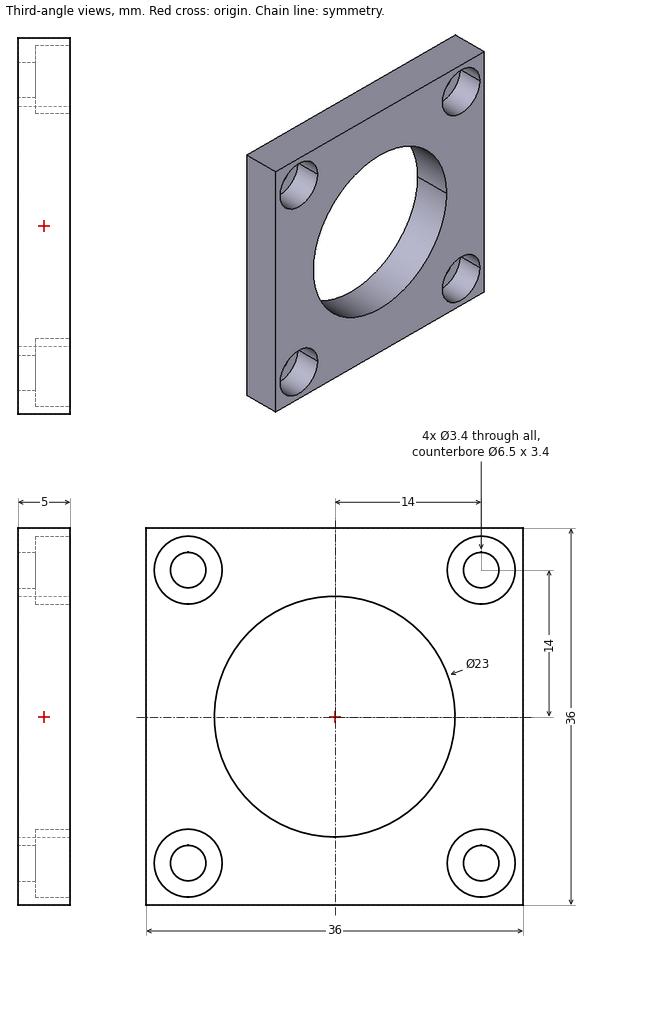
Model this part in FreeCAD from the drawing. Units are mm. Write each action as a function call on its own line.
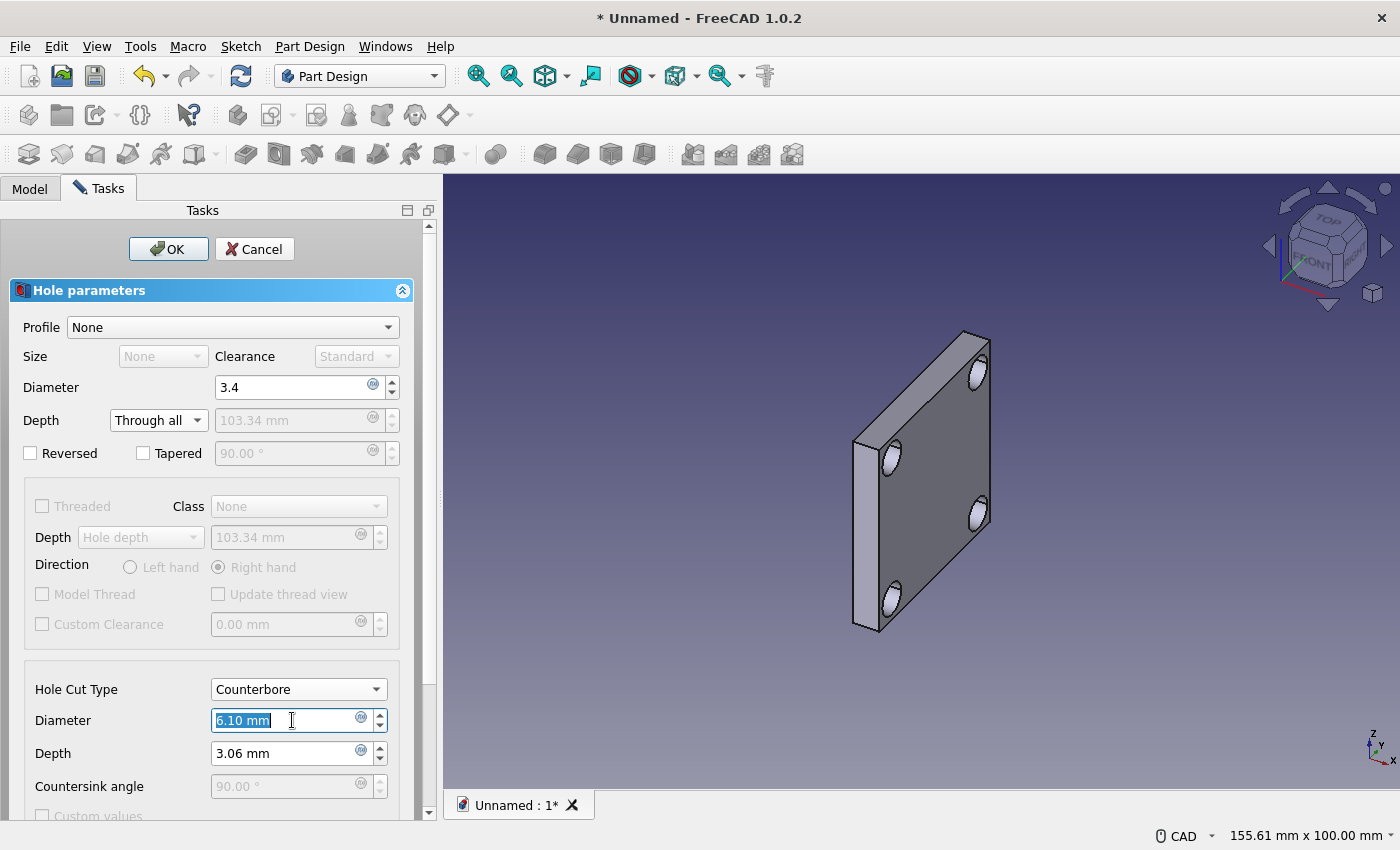
text(6.5)
key(Tab)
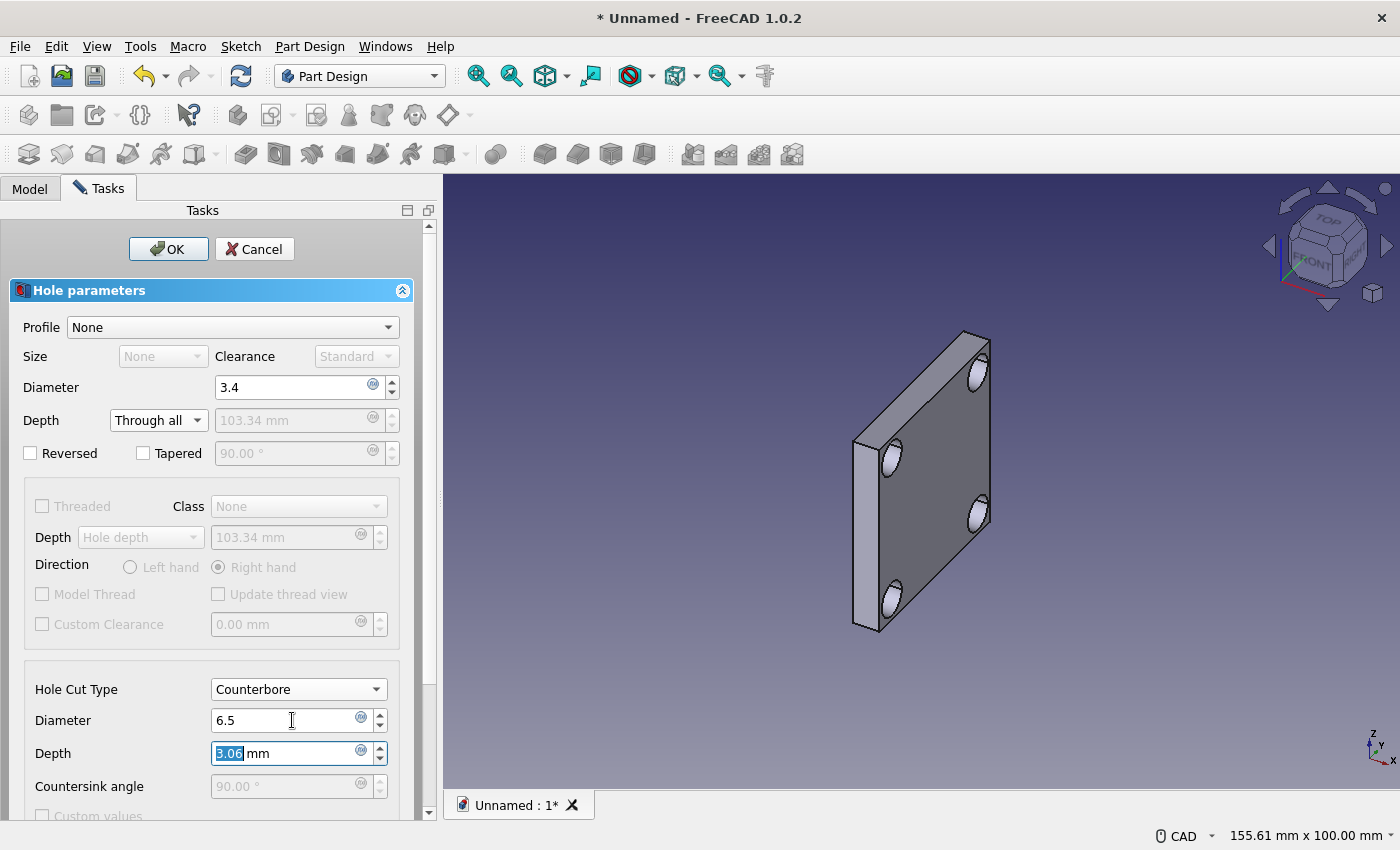
text(3.4)
key(Tab)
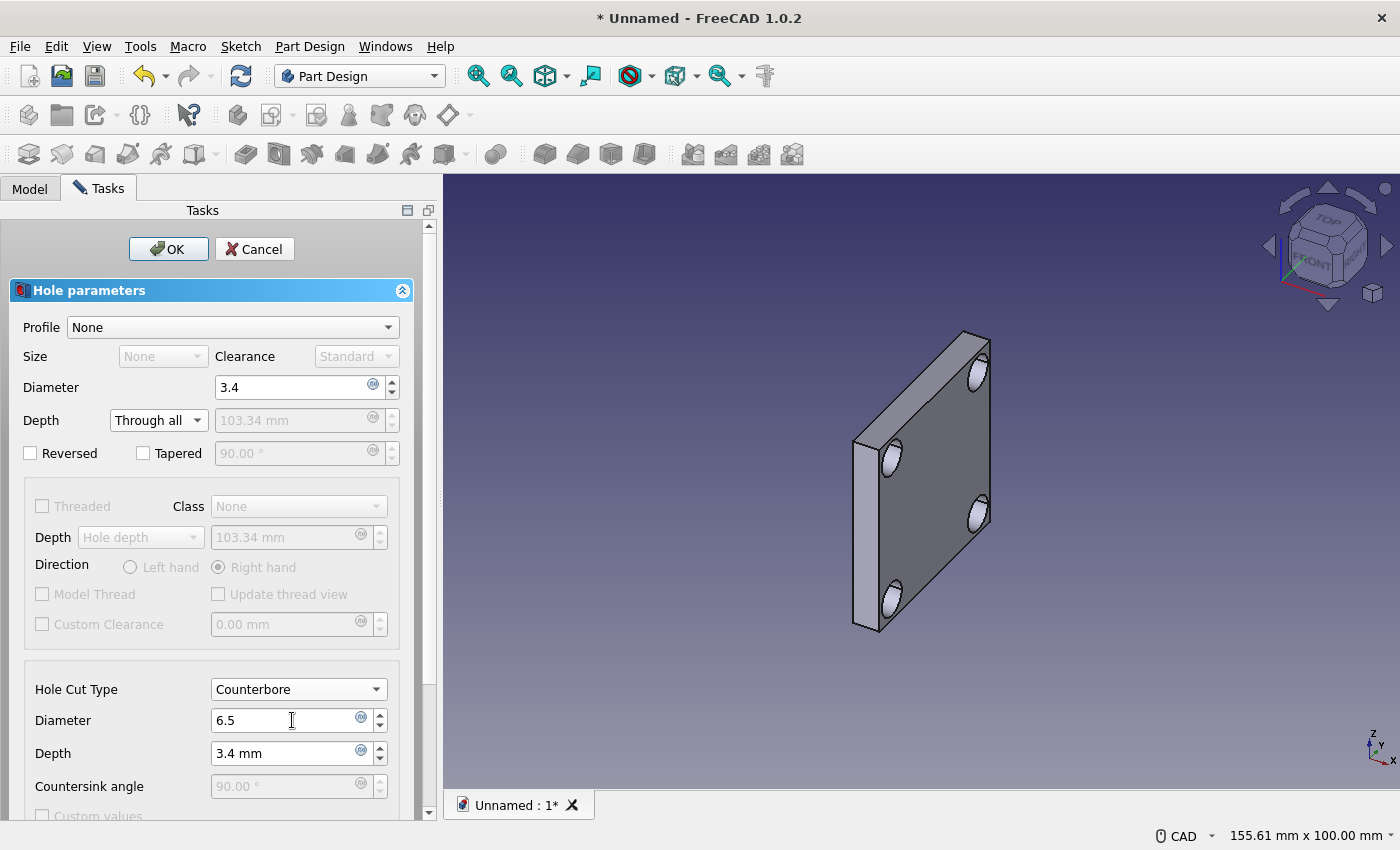
click(169, 249)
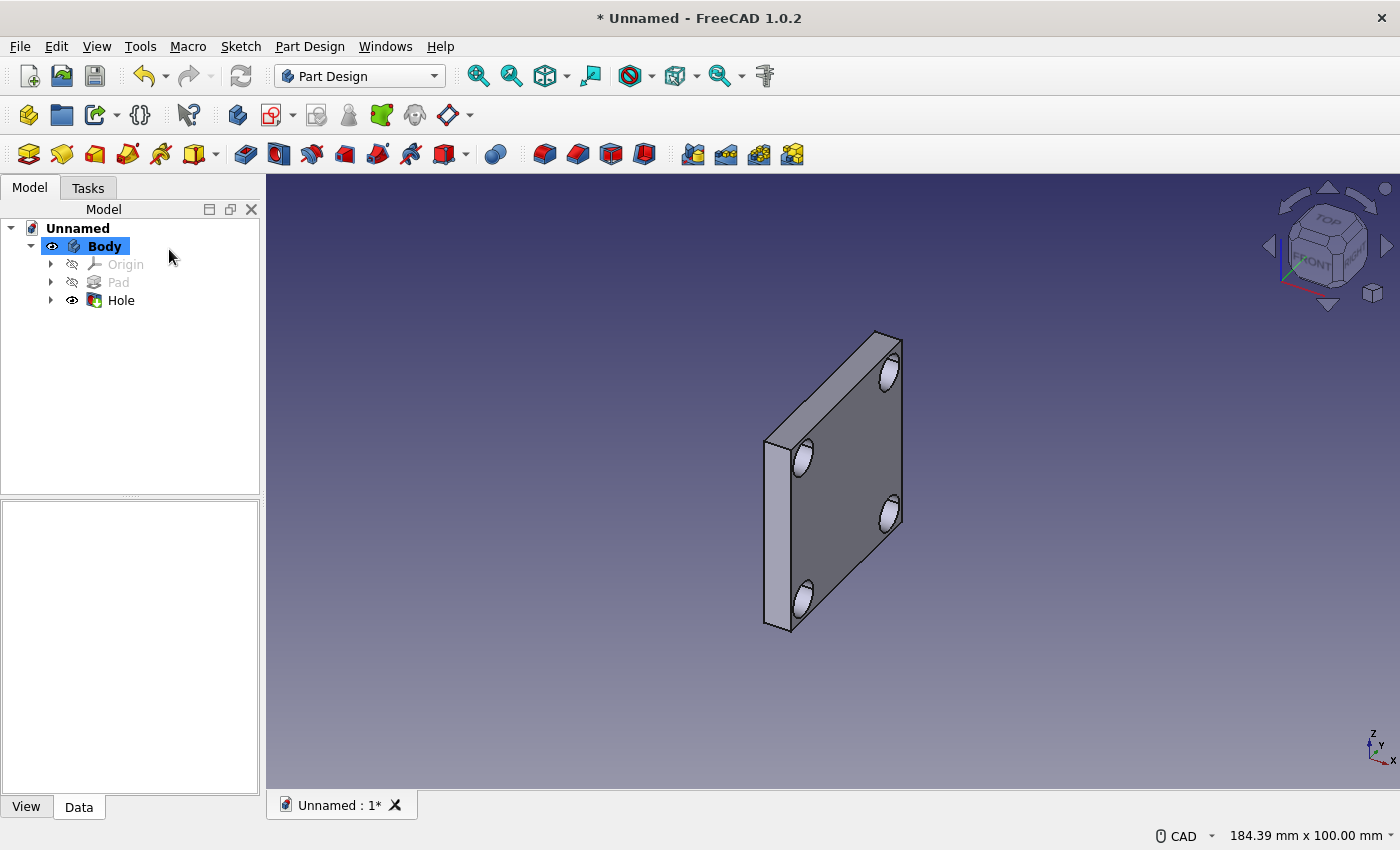
click(846, 485)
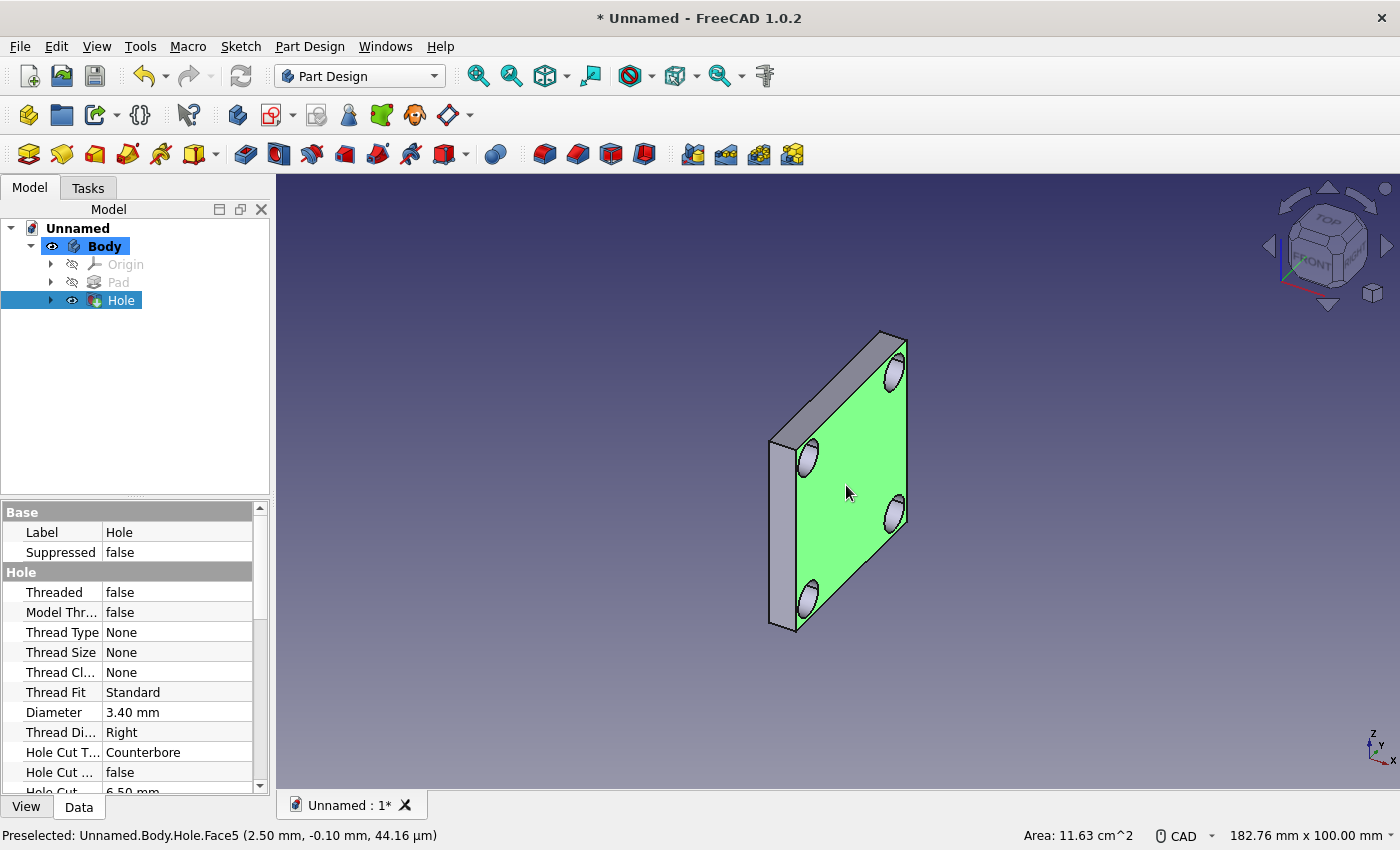
click(270, 116)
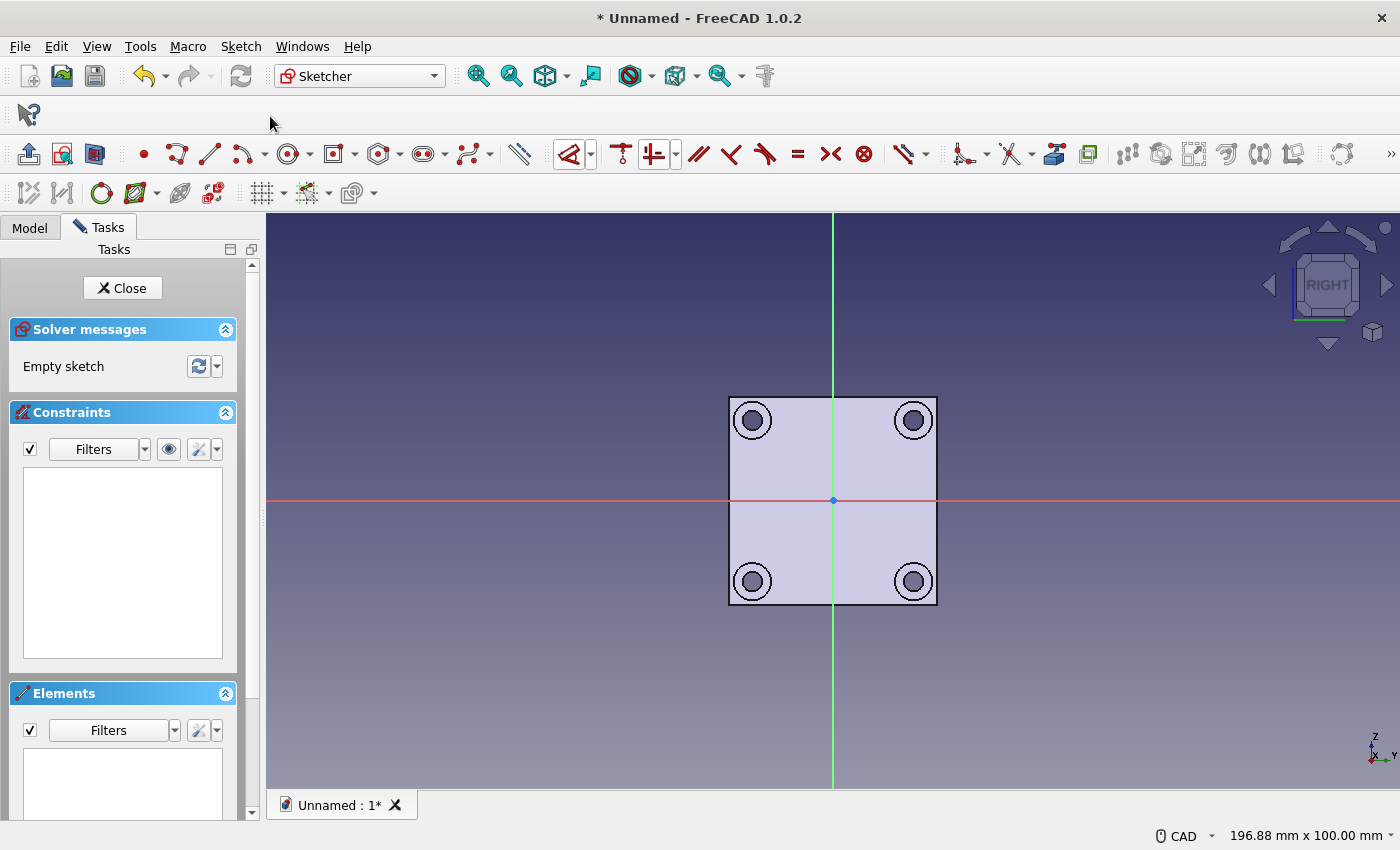
scroll(873, 501, up, 5)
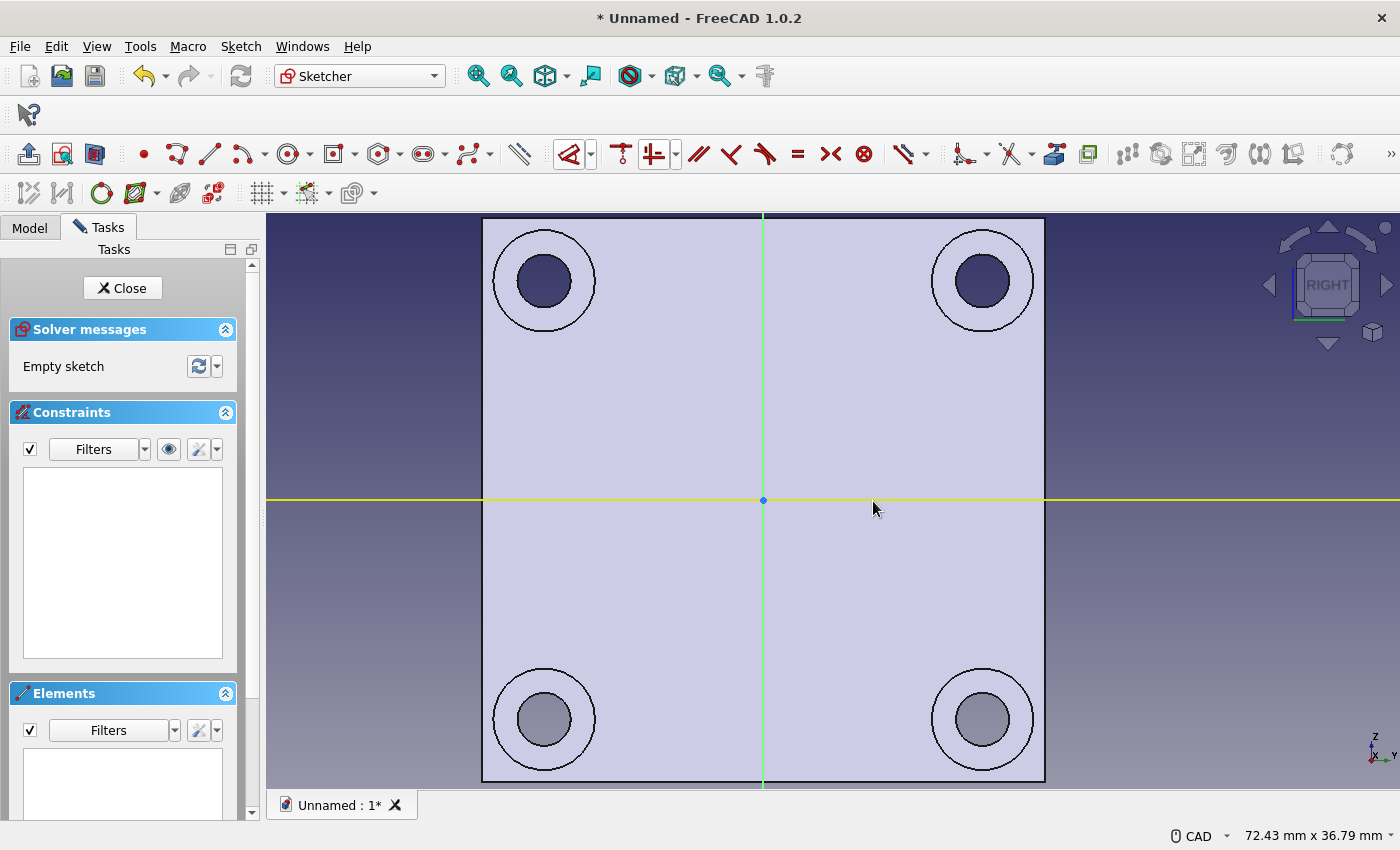
click(288, 154)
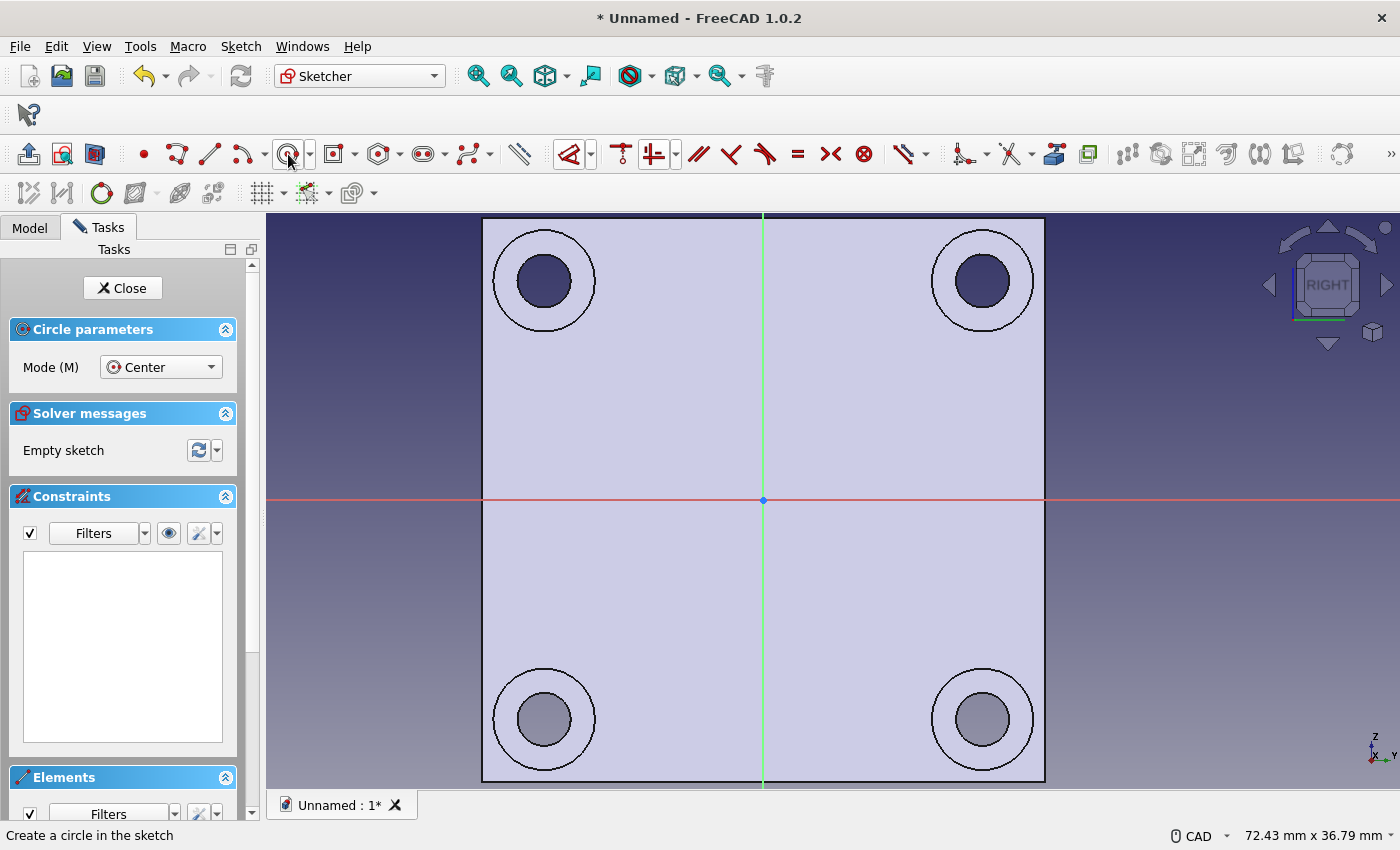
click(763, 500)
click(891, 373)
key(Escape)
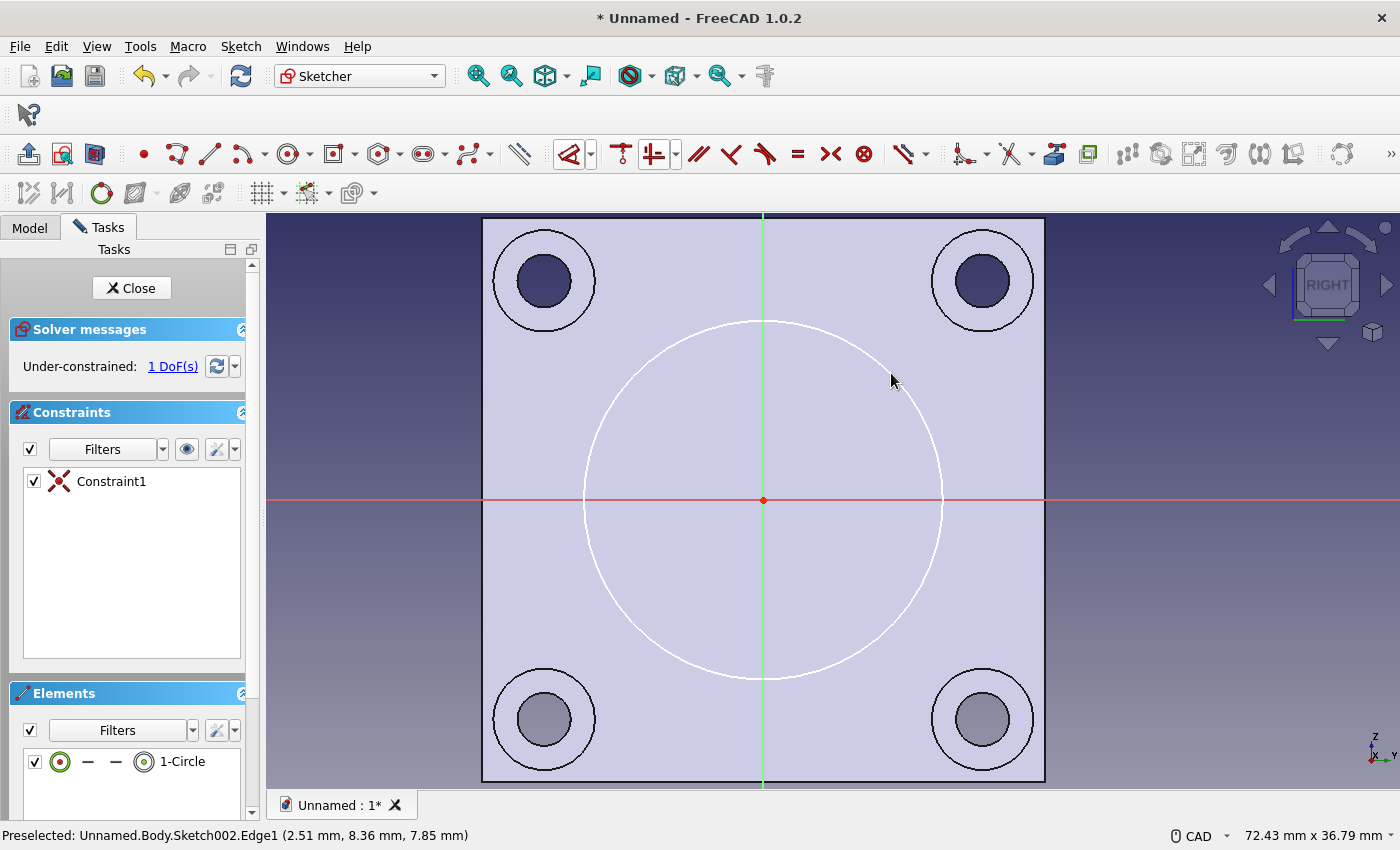
click(890, 373)